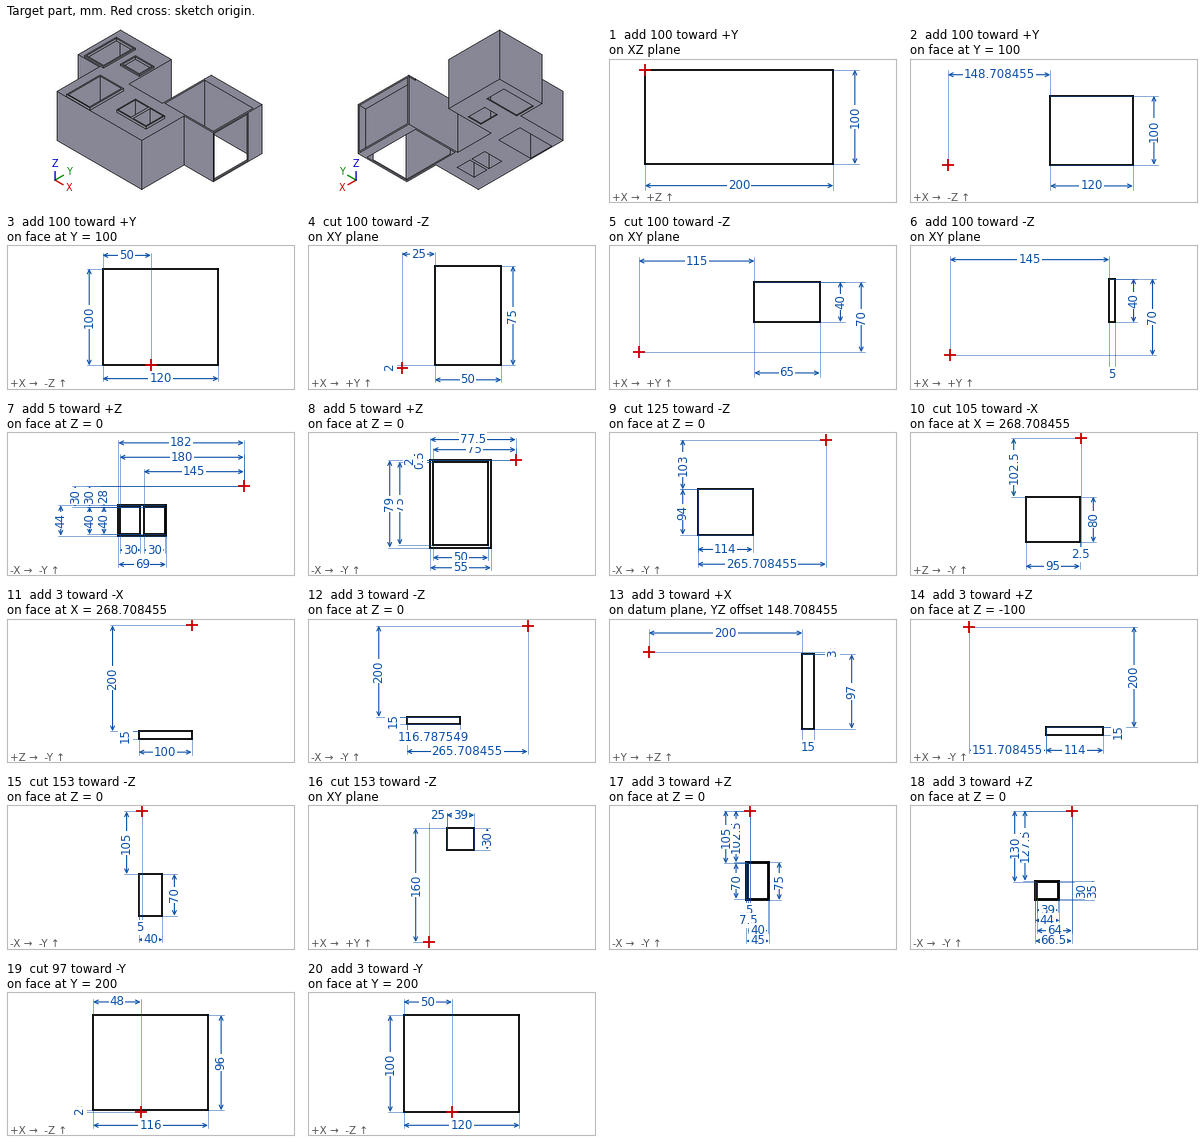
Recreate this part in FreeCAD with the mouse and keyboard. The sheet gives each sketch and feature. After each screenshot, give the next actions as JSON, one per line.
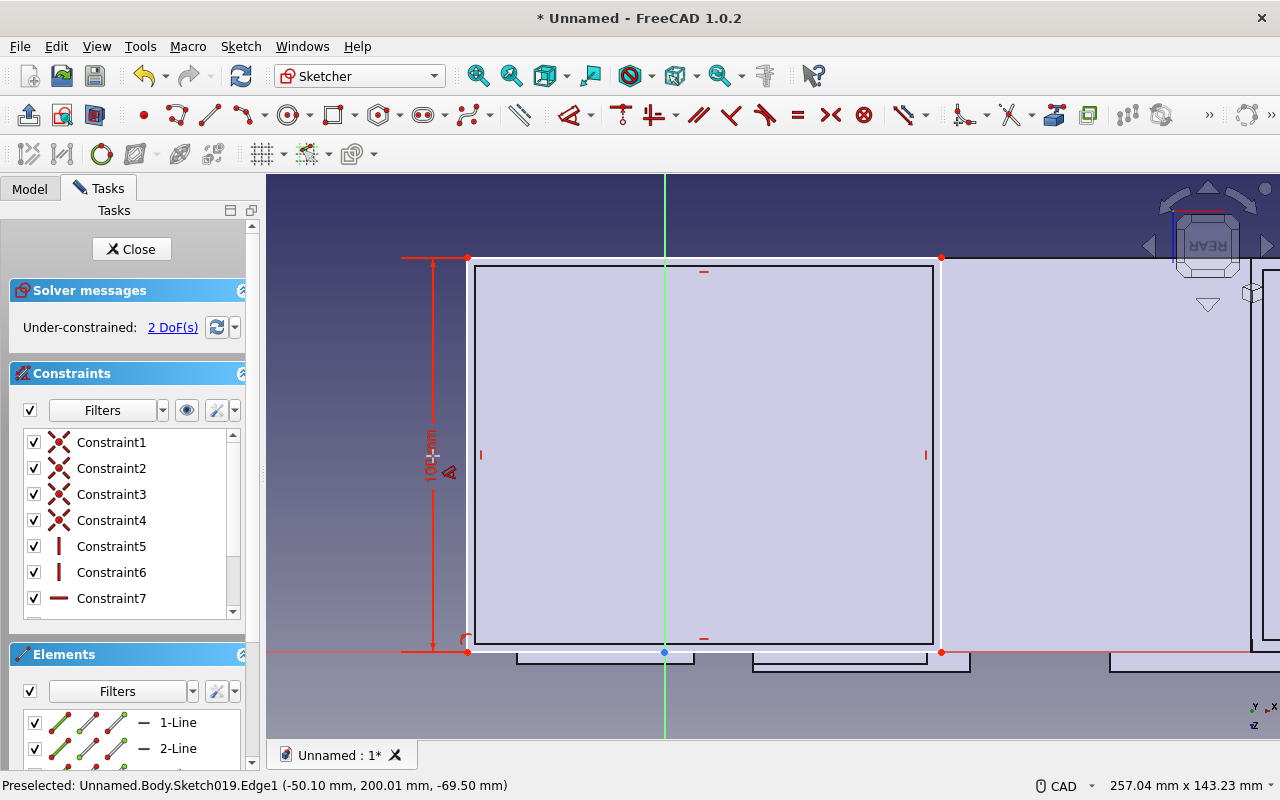
{"action": "left_click", "coordinate": [609, 652]}
{"action": "left_click", "coordinate": [704, 686]}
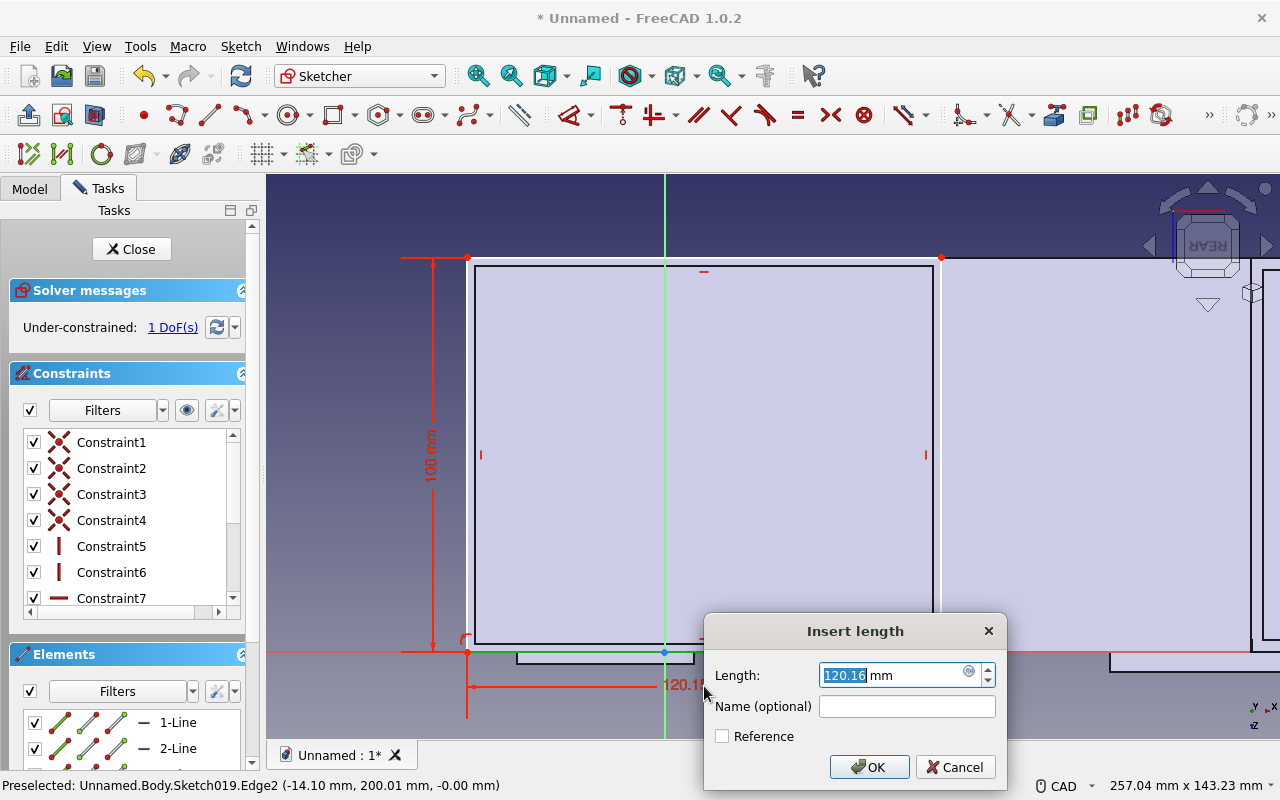
{"action": "type", "text": "120"}
{"action": "key", "text": "Return"}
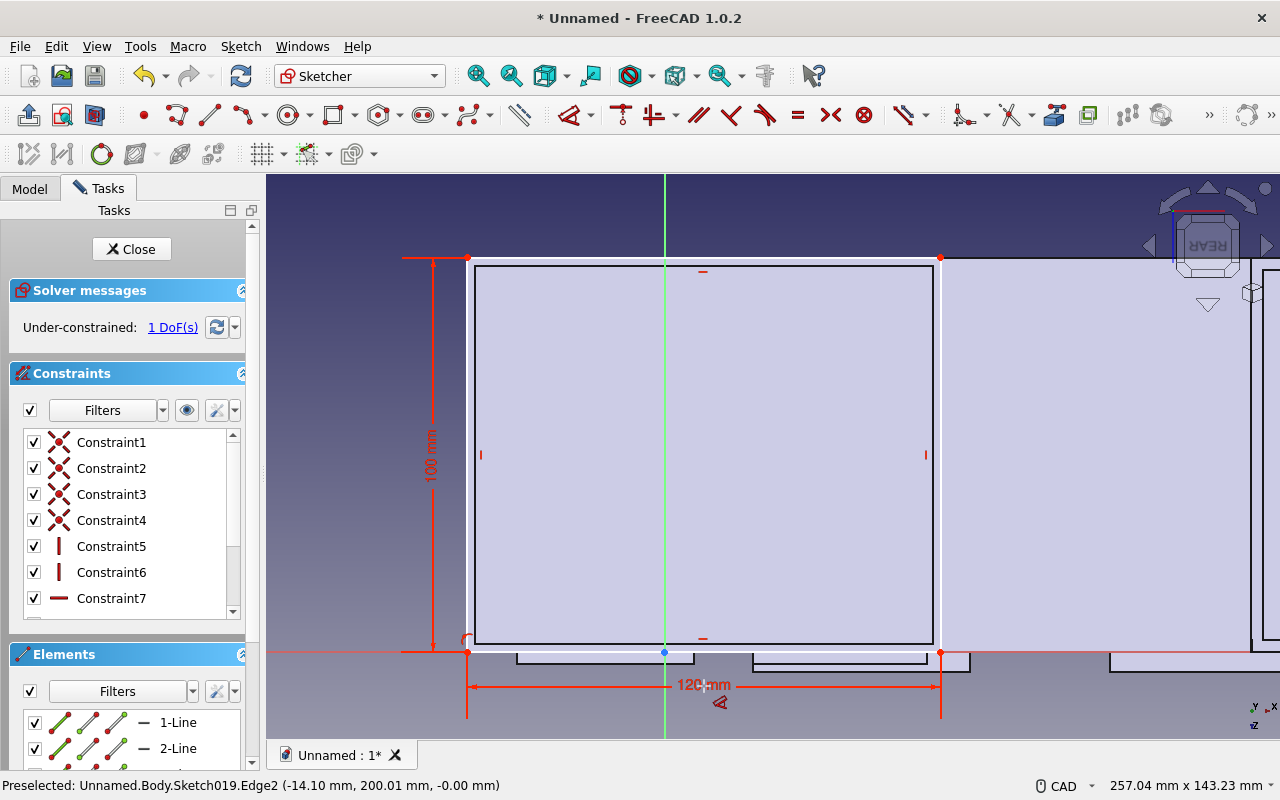
{"action": "left_click", "coordinate": [467, 258]}
{"action": "left_click", "coordinate": [566, 686]}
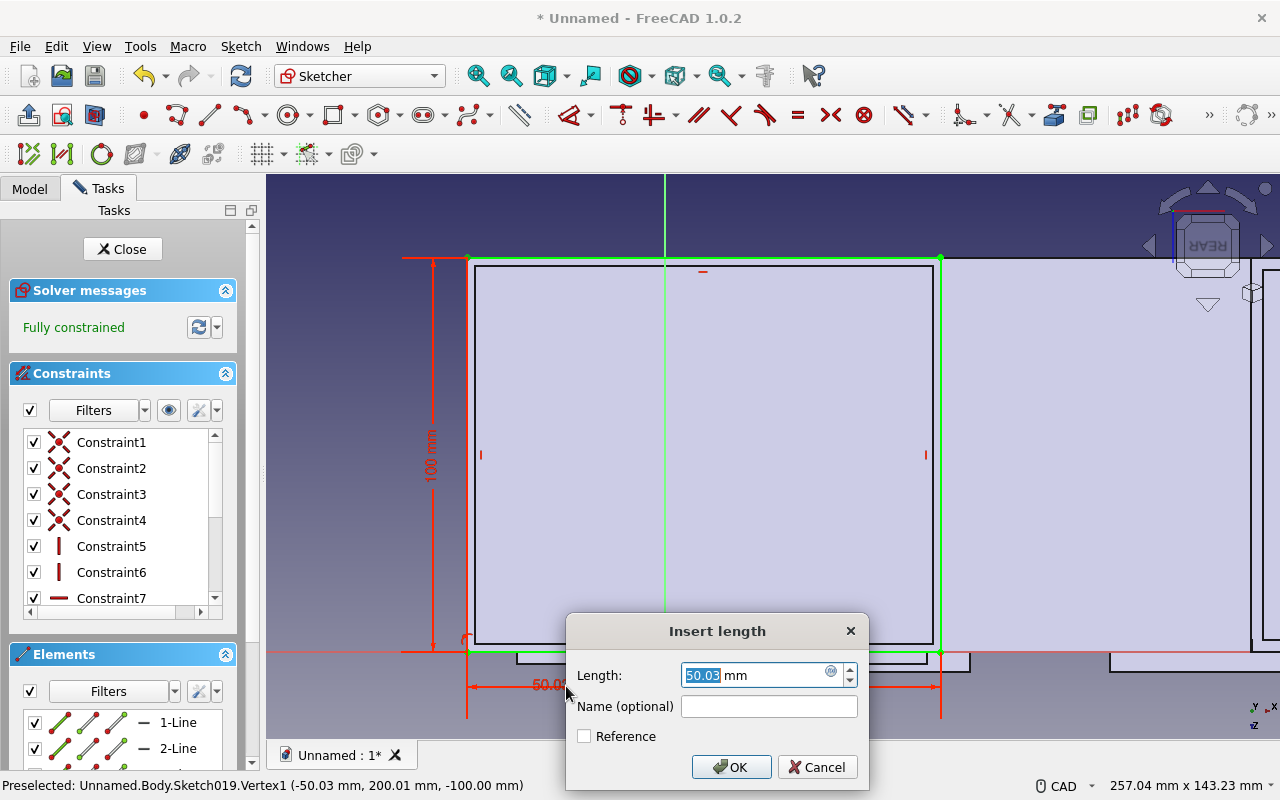
{"action": "type", "text": "50"}
{"action": "key", "text": "Return"}
{"action": "key", "text": "Escape"}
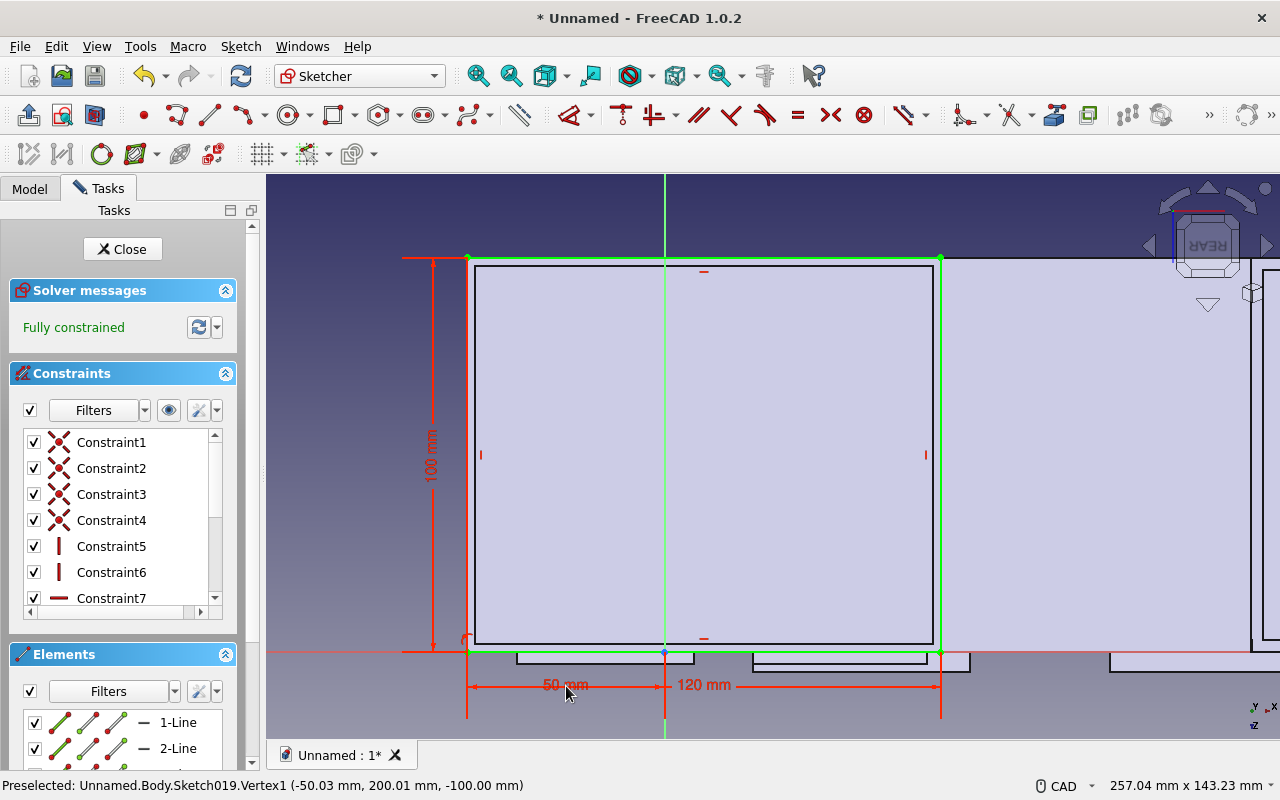
{"action": "left_click", "coordinate": [123, 249]}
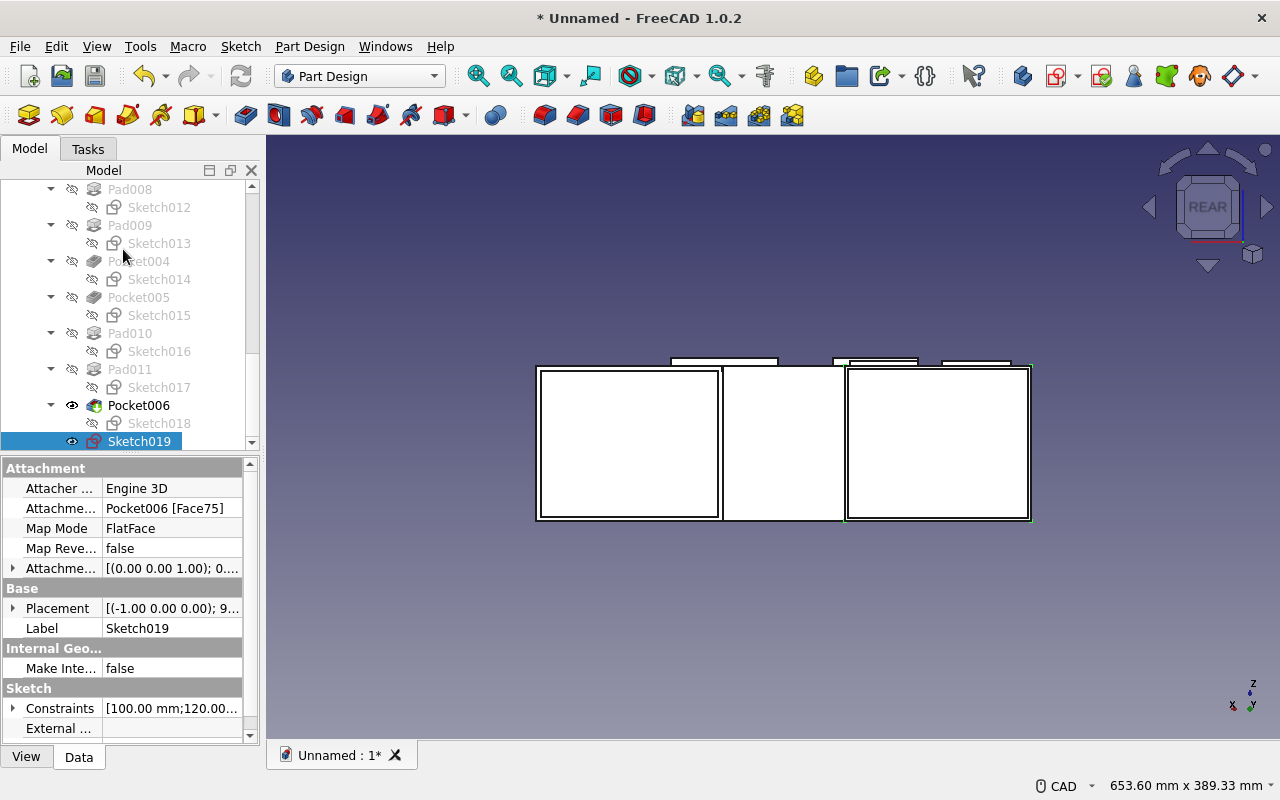
{"action": "left_click", "coordinate": [29, 116]}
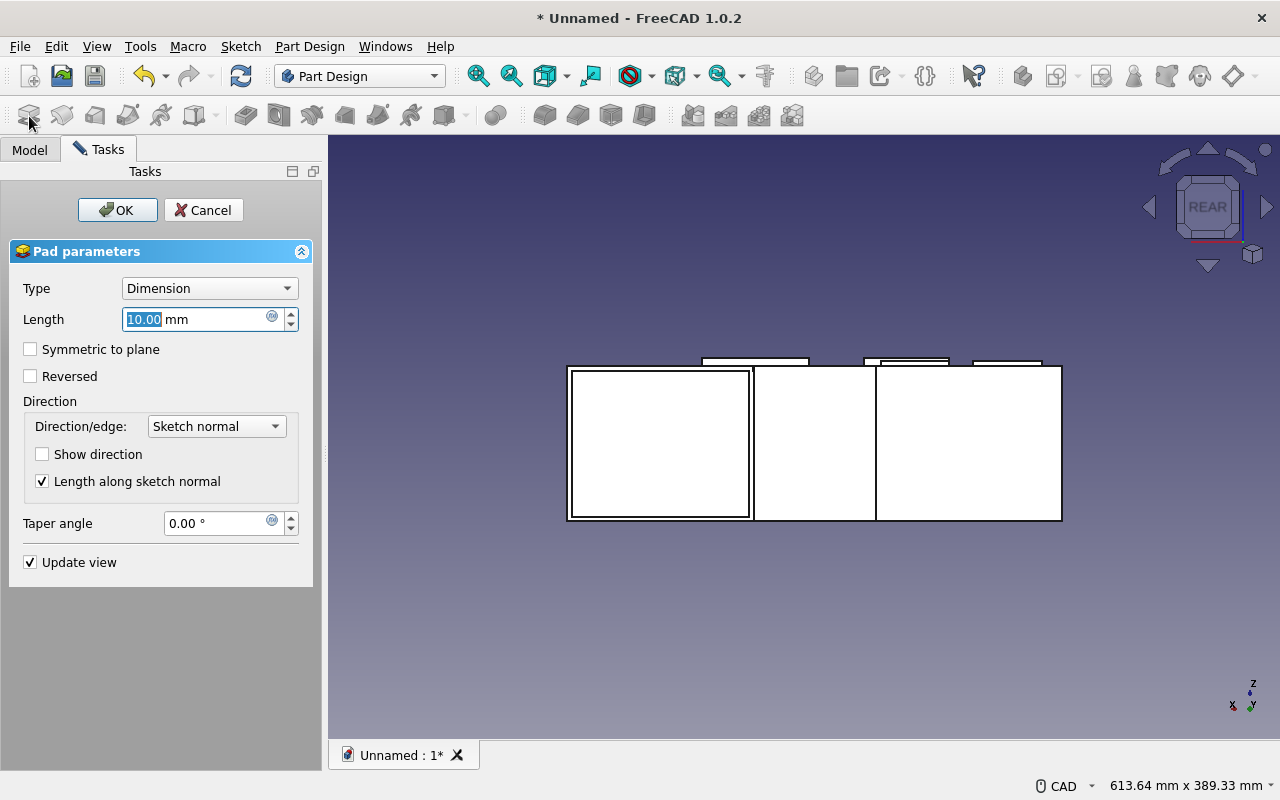
{"action": "type", "text": "3"}
{"action": "key", "text": "Tab"}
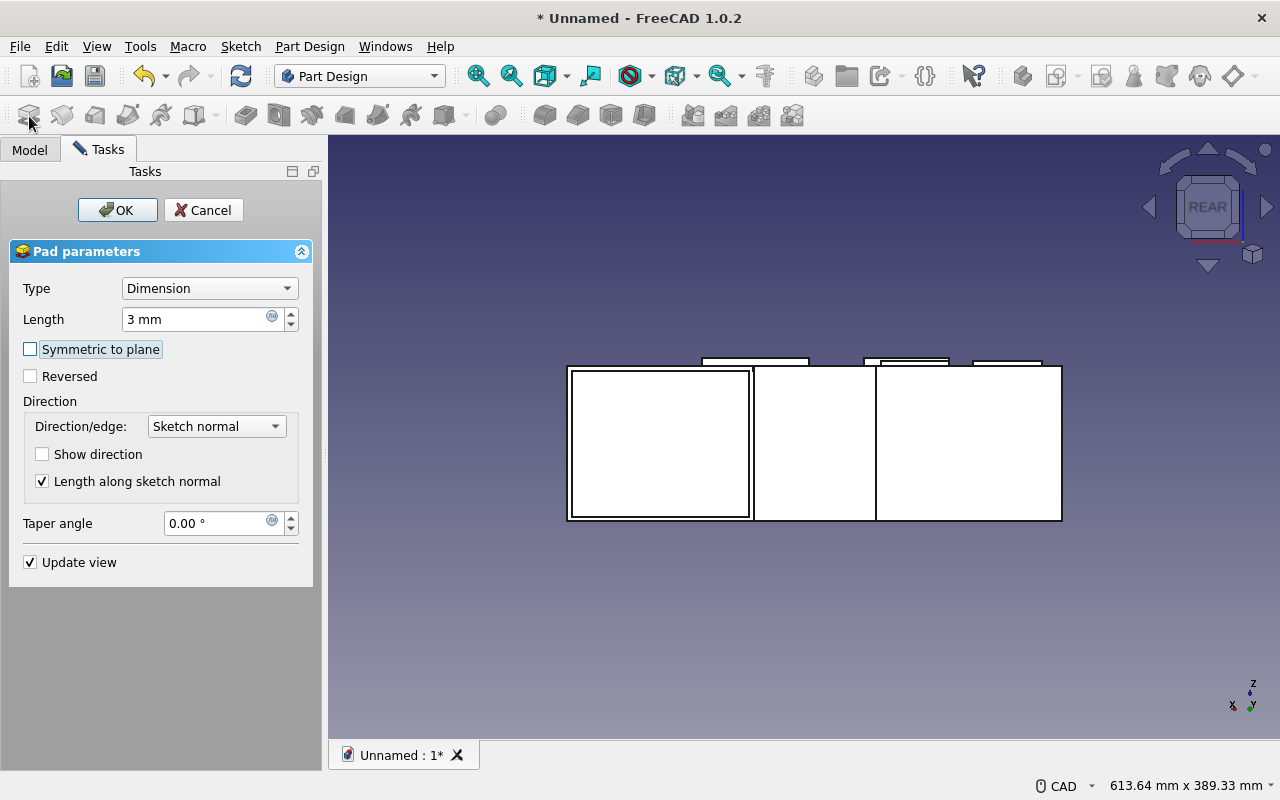
{"action": "left_click", "coordinate": [31, 376]}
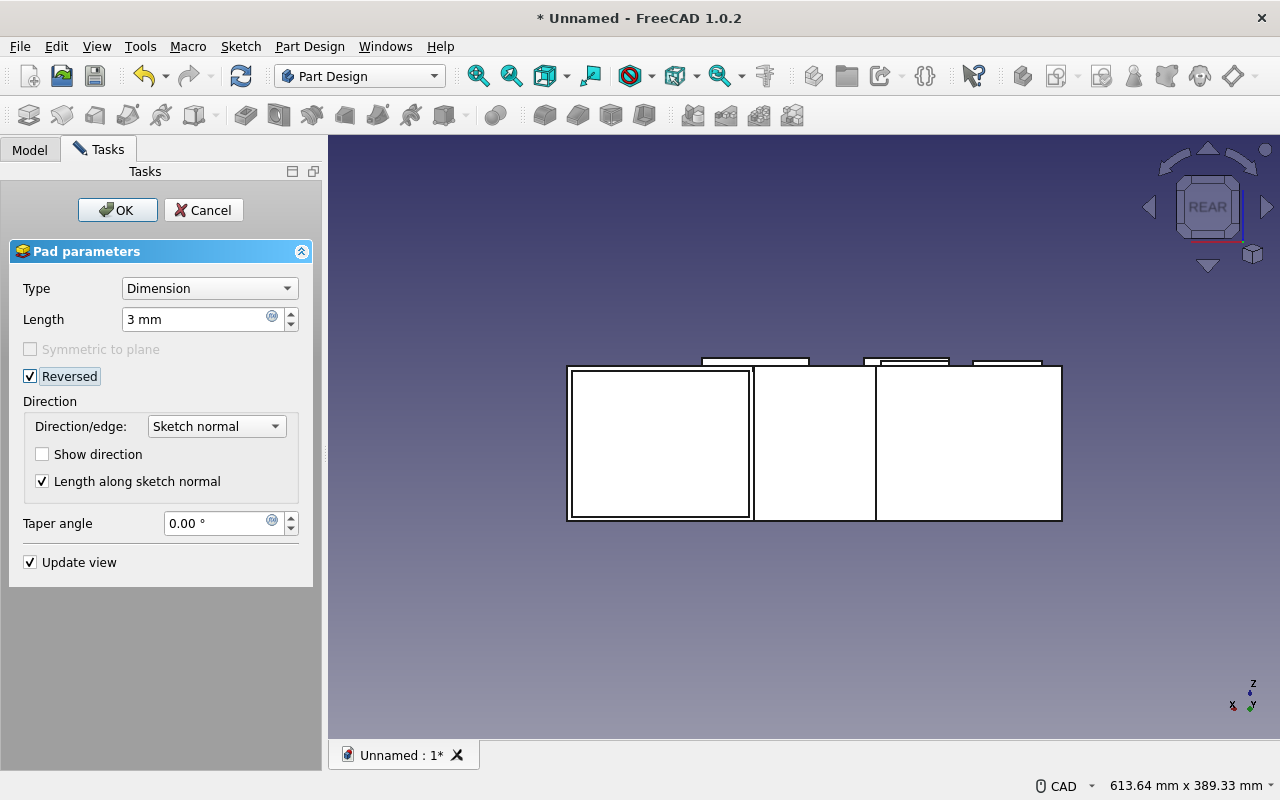
{"action": "left_click", "coordinate": [118, 210]}